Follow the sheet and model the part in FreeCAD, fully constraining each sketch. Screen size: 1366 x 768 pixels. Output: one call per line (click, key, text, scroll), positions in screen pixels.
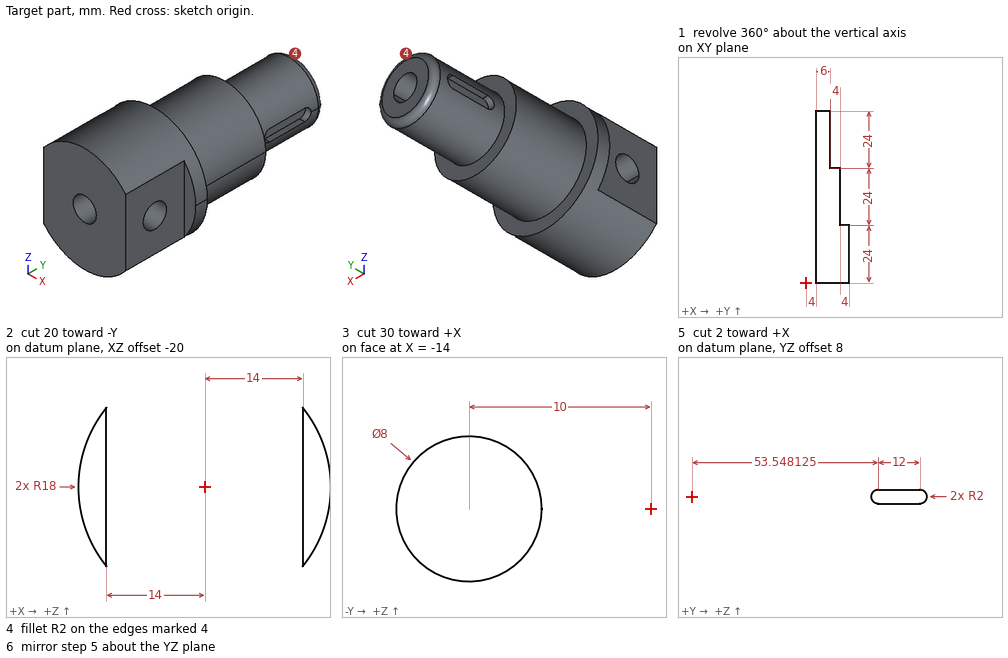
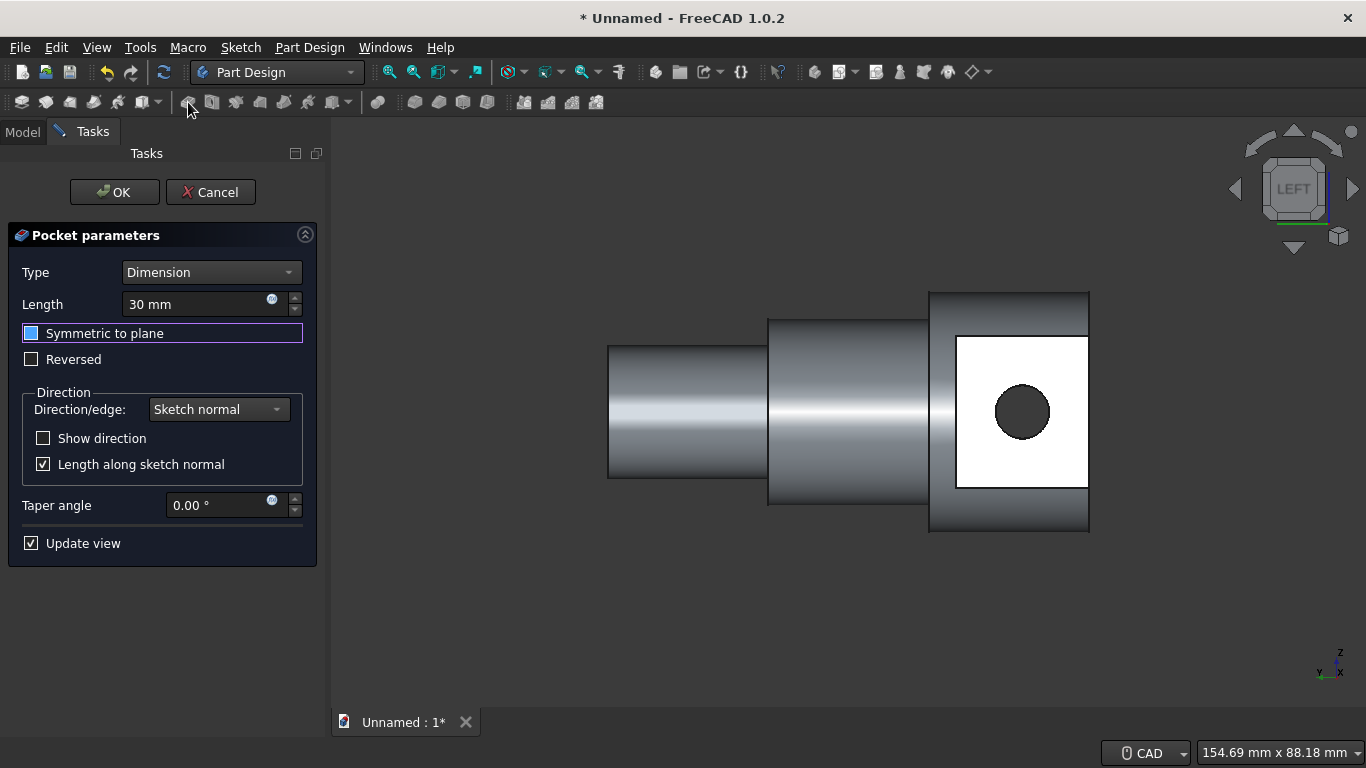
click(115, 192)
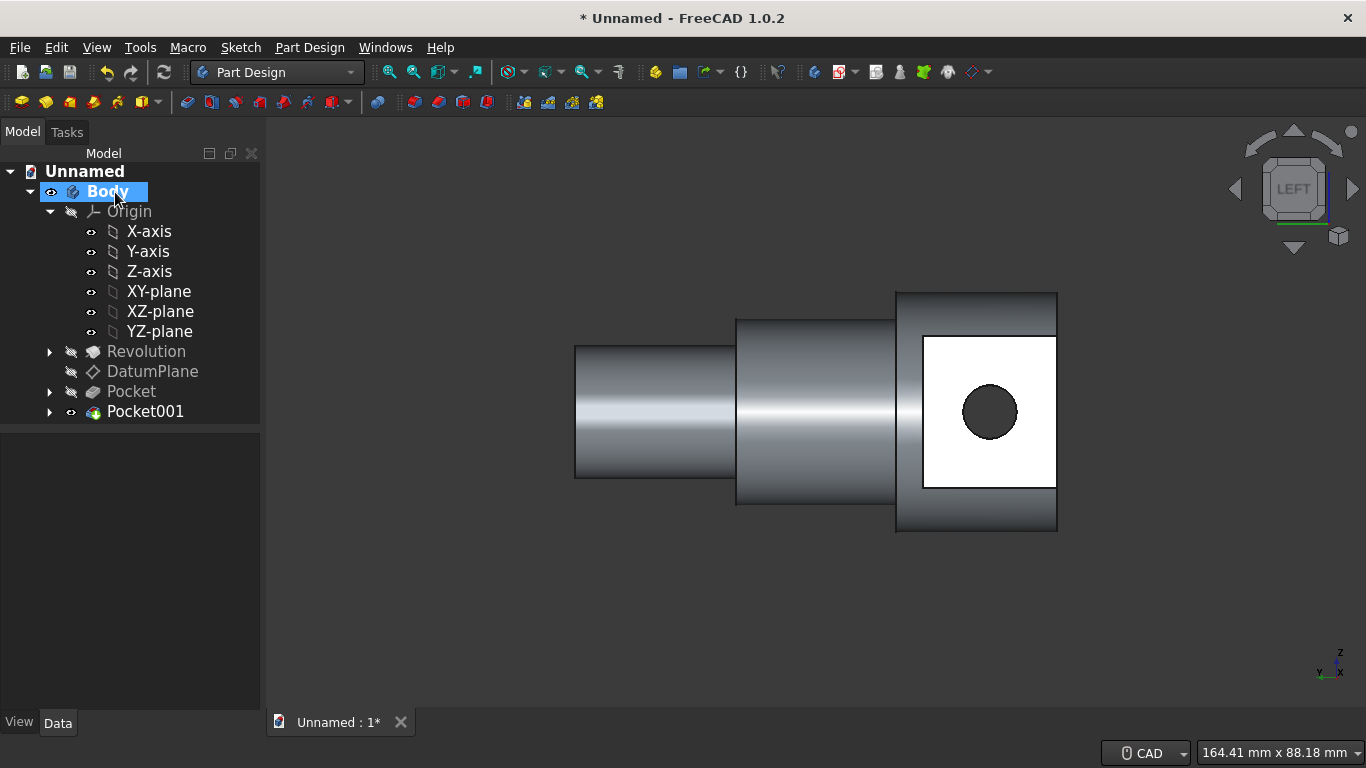
click(390, 72)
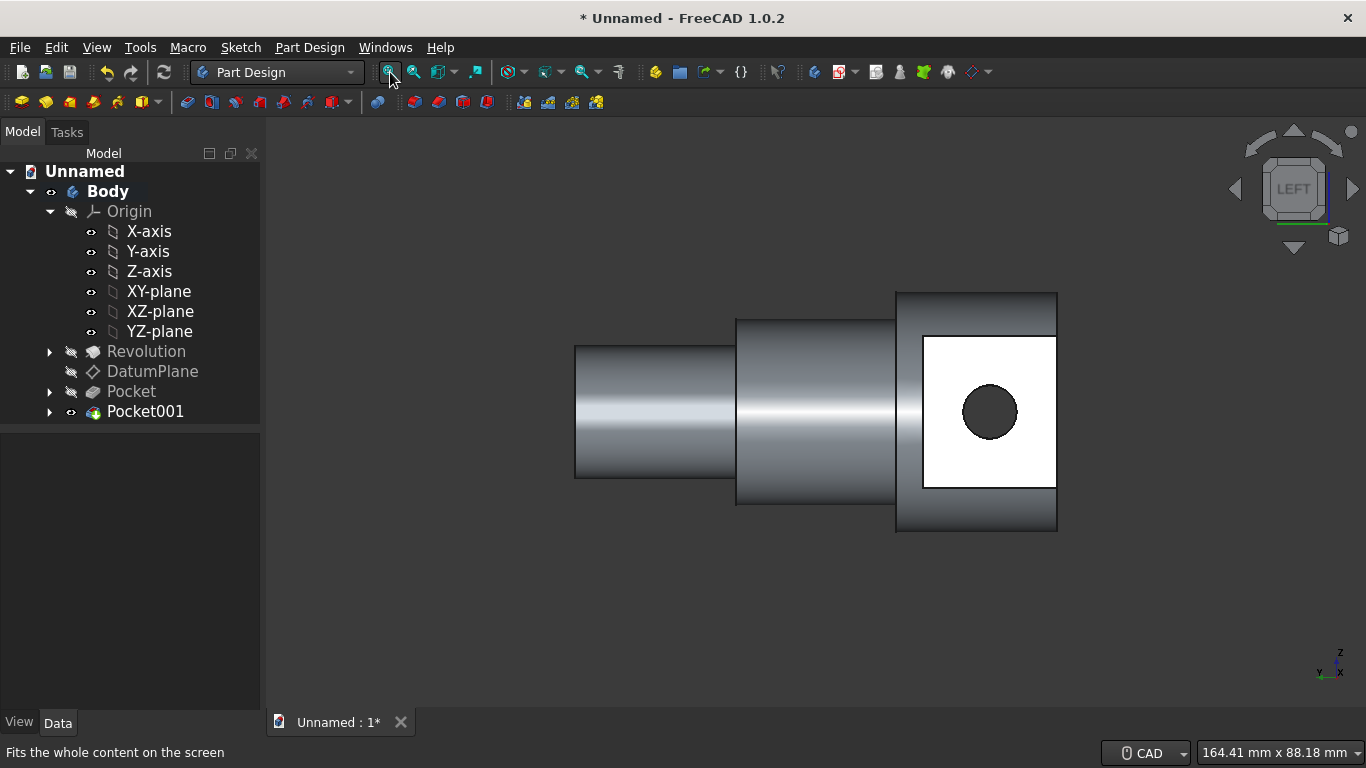
click(575, 411)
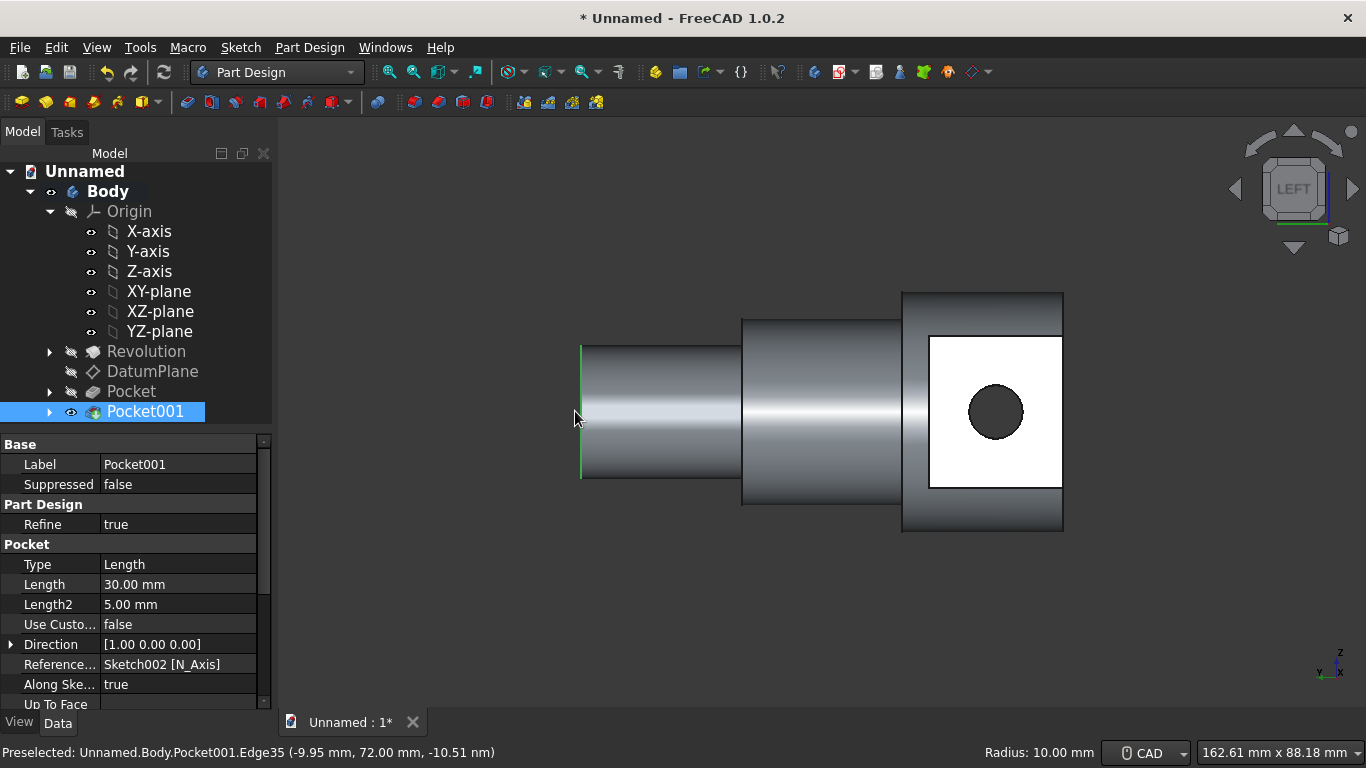
click(416, 102)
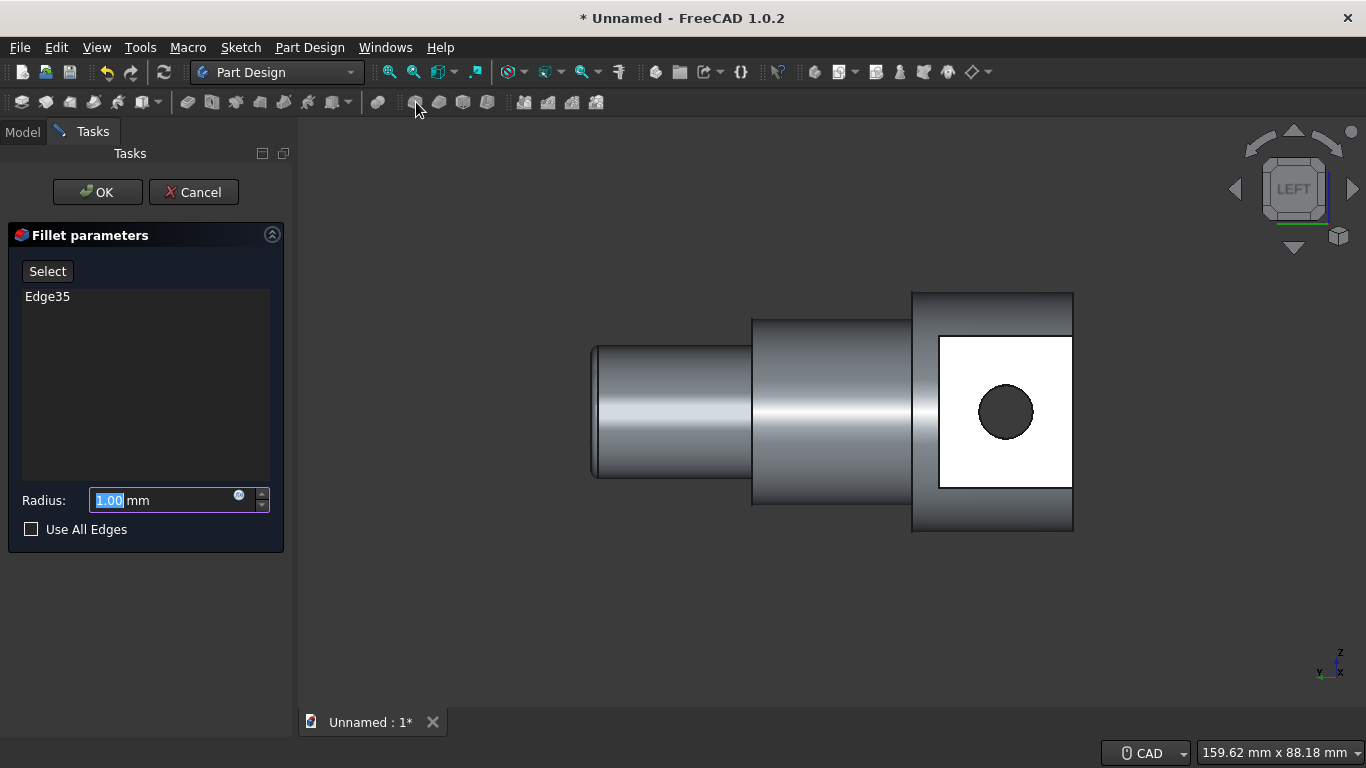
text(2)
key(Tab)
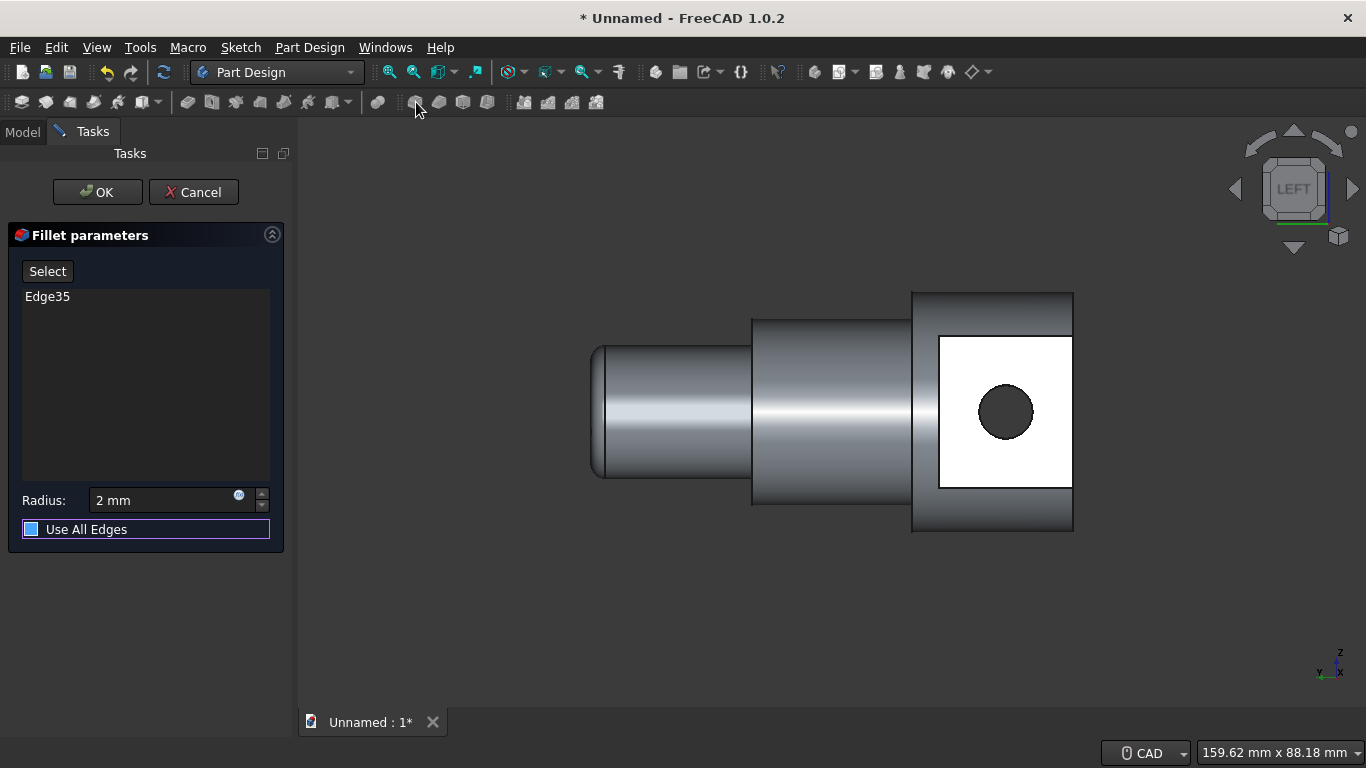
click(98, 192)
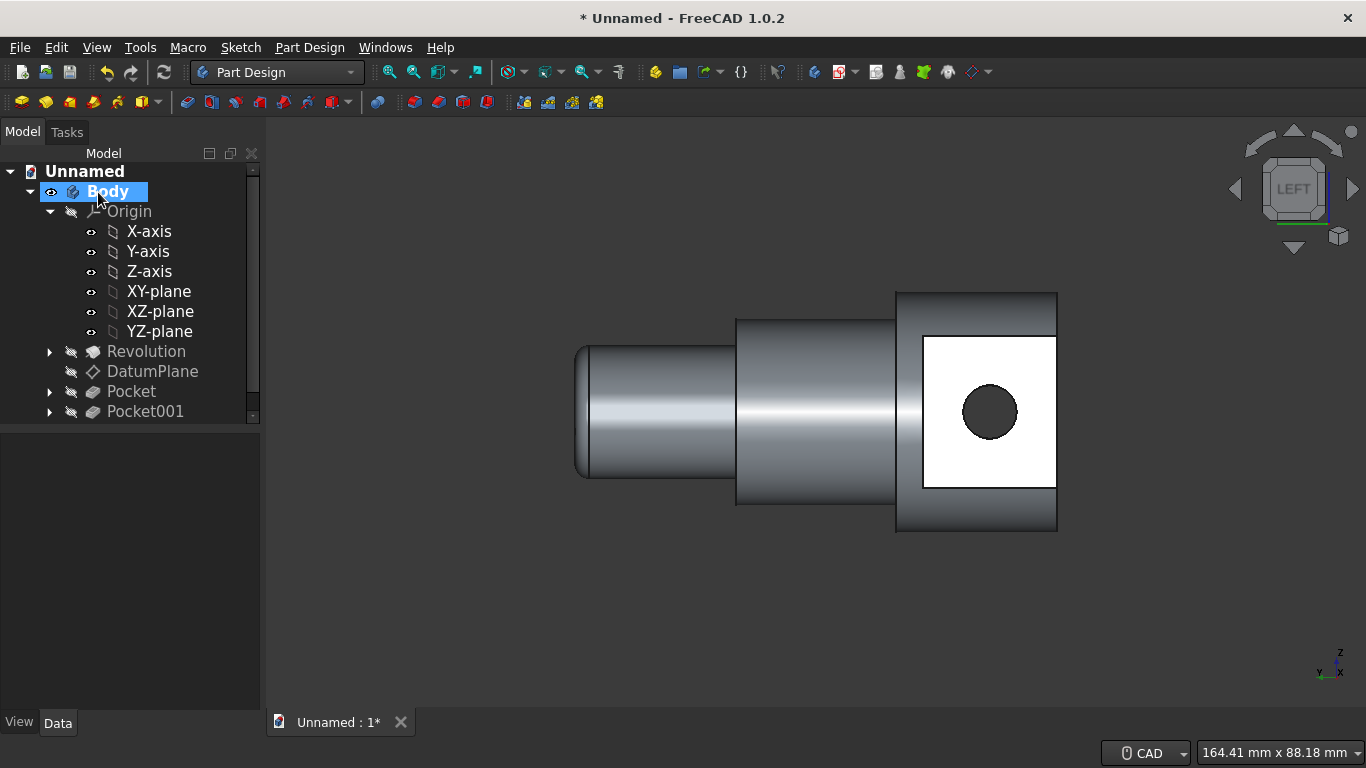
click(390, 72)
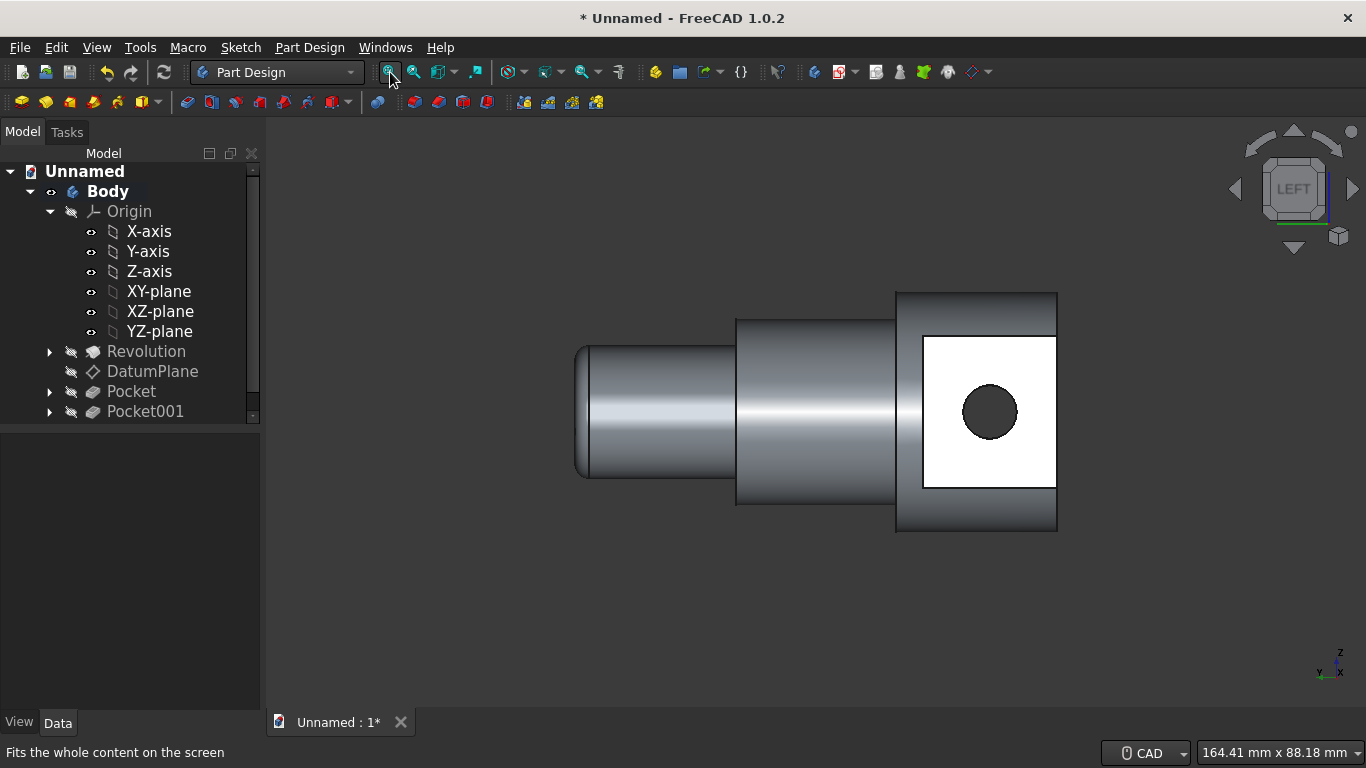
click(136, 332)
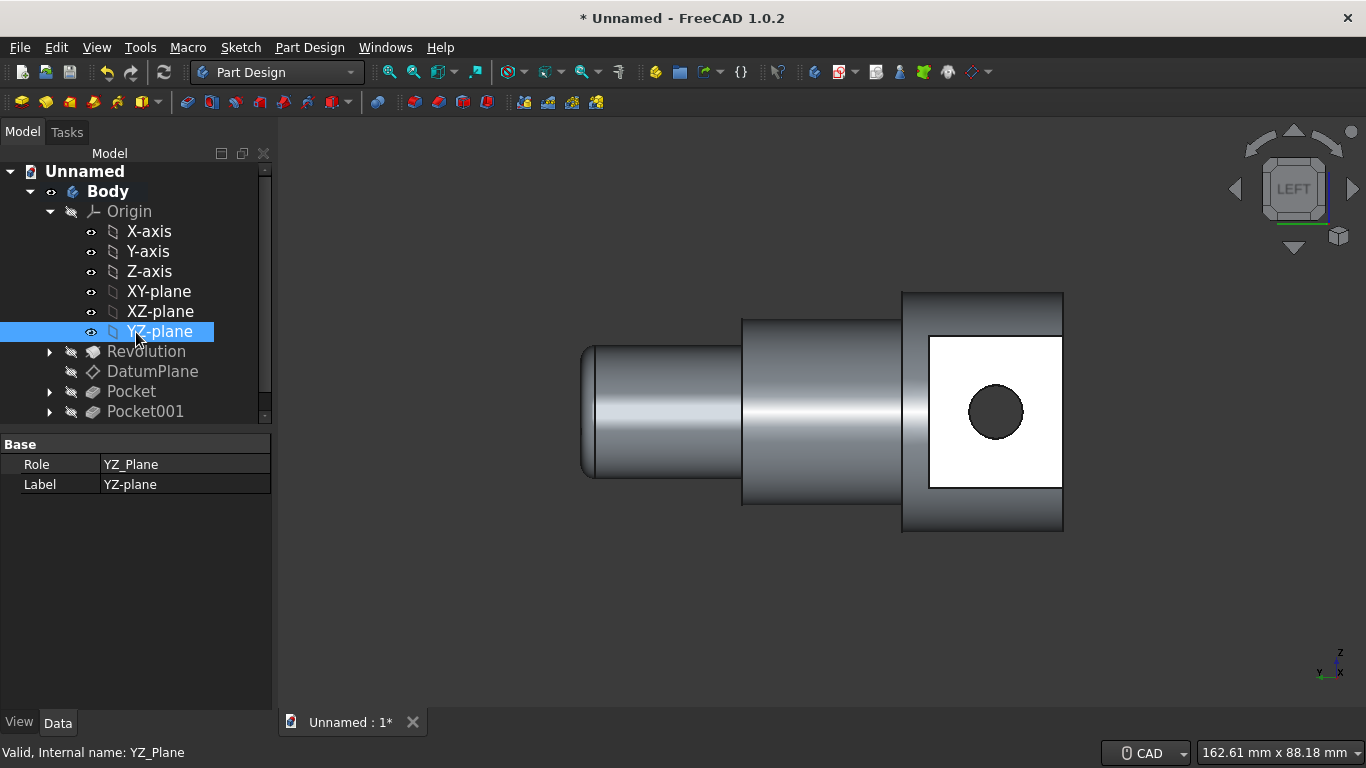
click(972, 72)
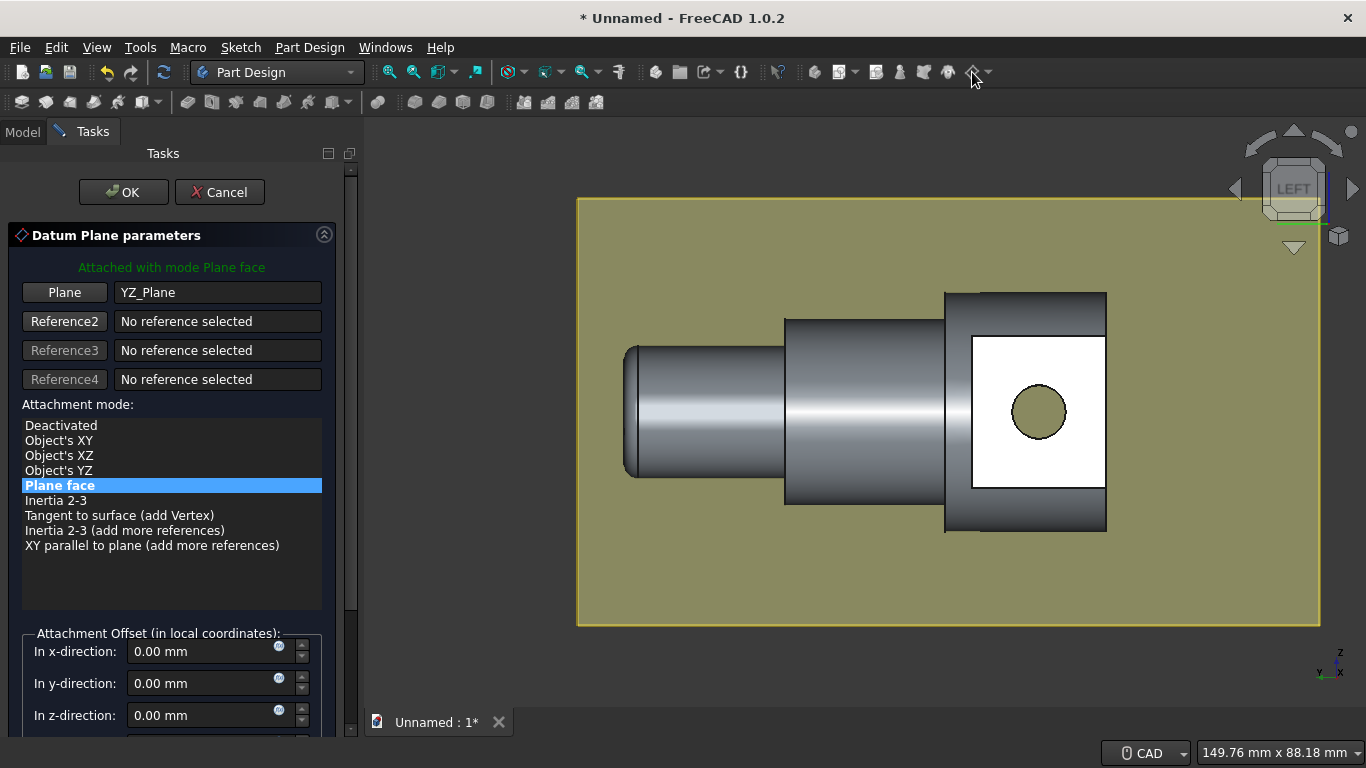
triple_click(210, 715)